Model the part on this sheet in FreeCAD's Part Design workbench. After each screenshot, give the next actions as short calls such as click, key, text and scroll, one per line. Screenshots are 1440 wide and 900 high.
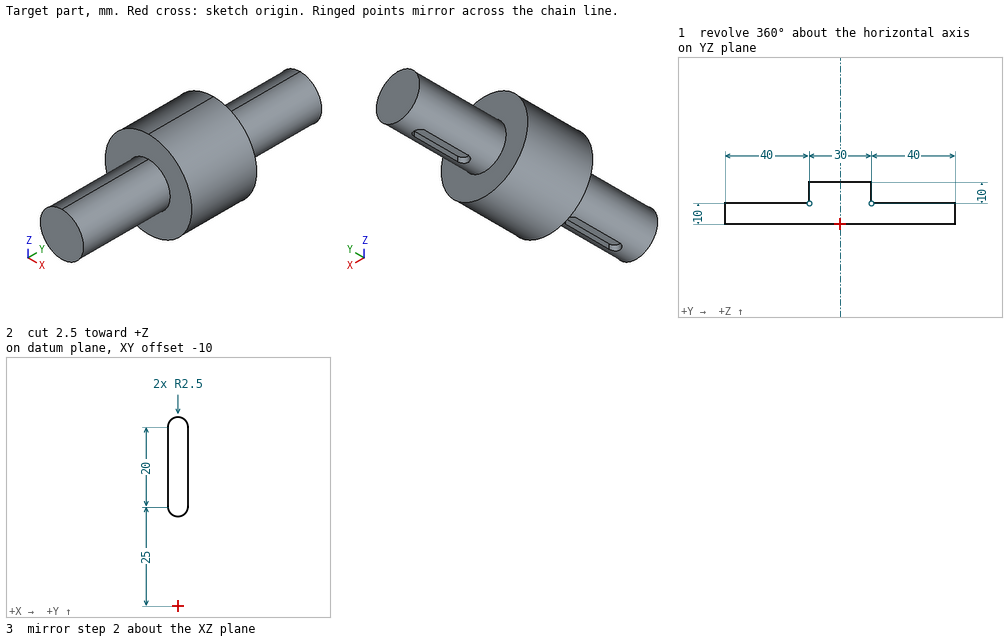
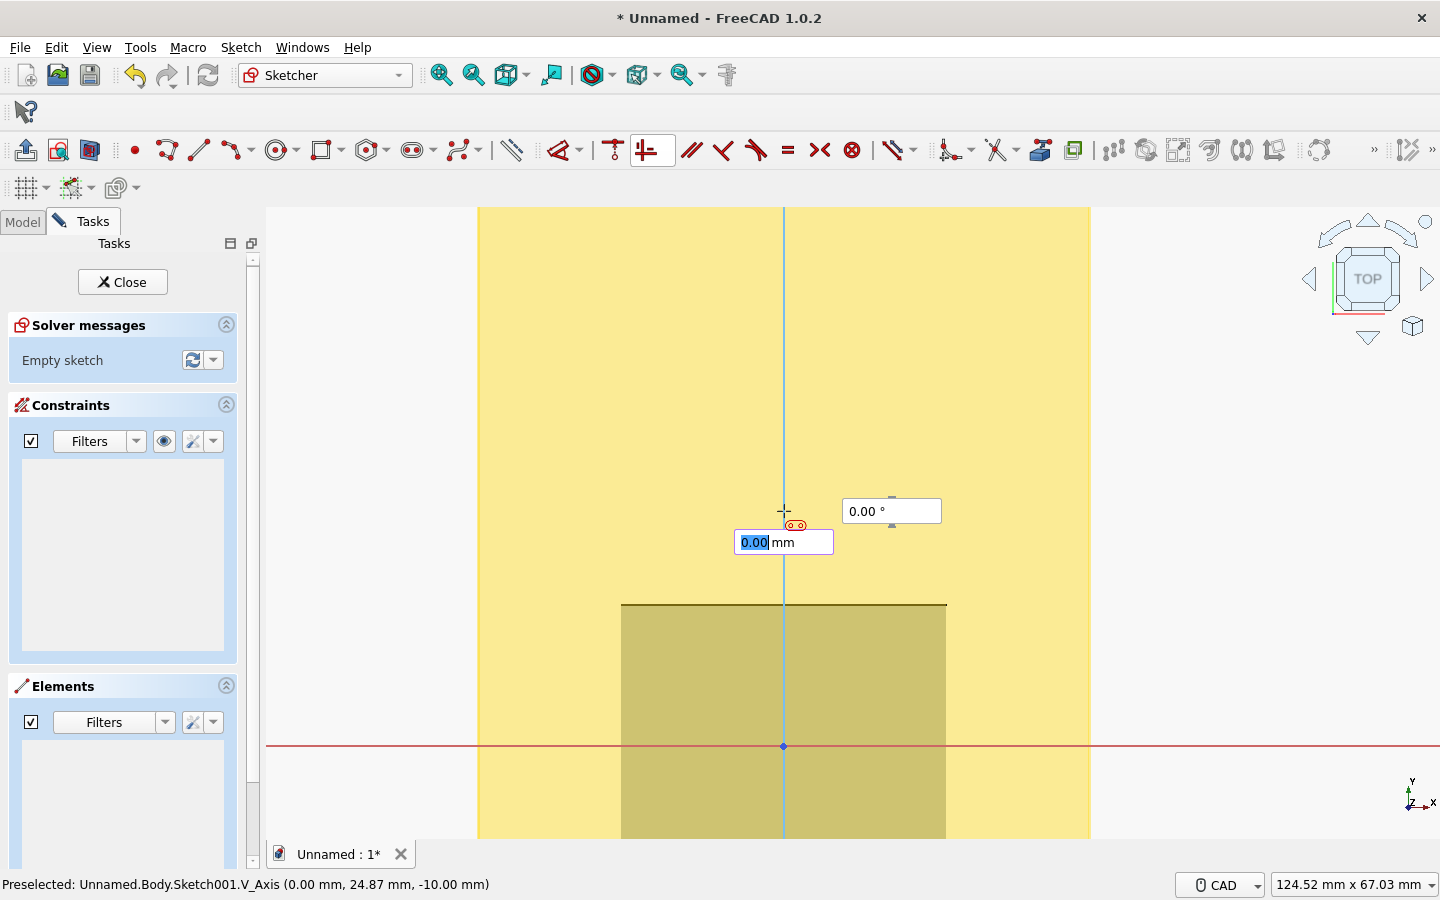
click(793, 322)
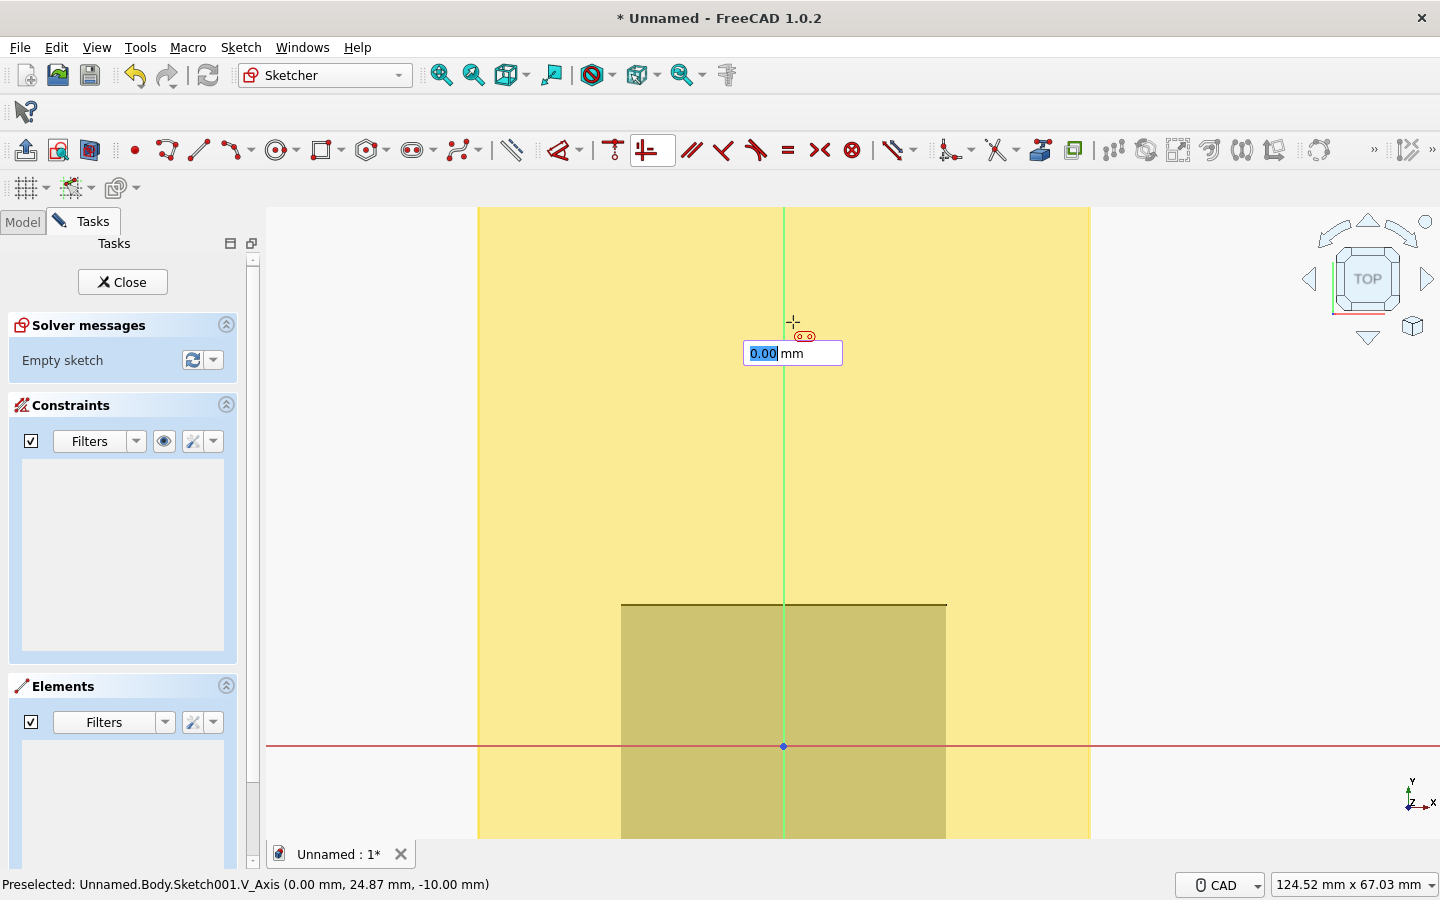
click(760, 416)
key(Escape)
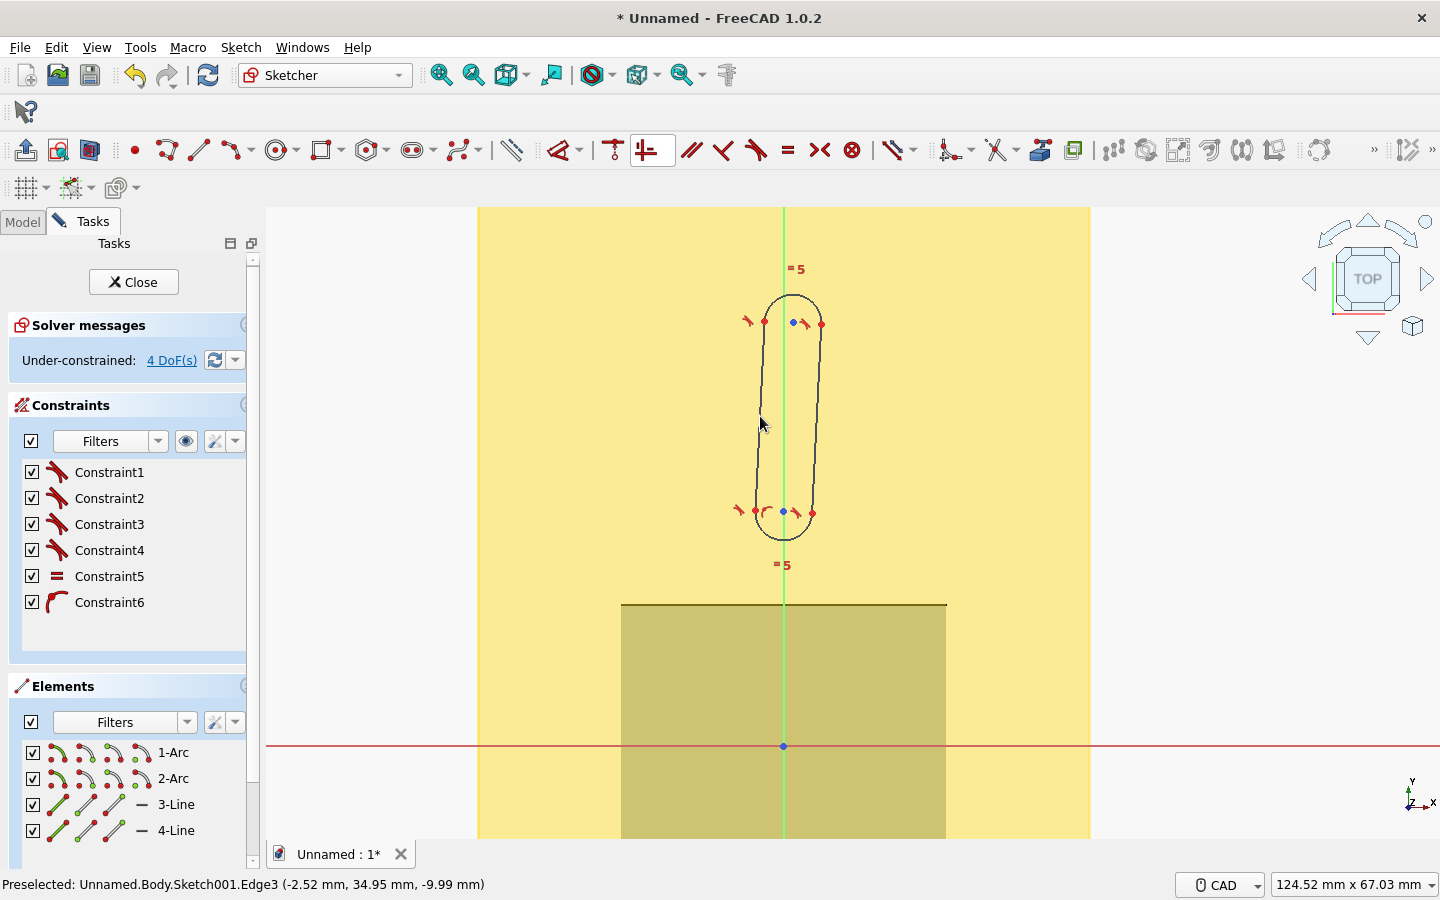
click(758, 454)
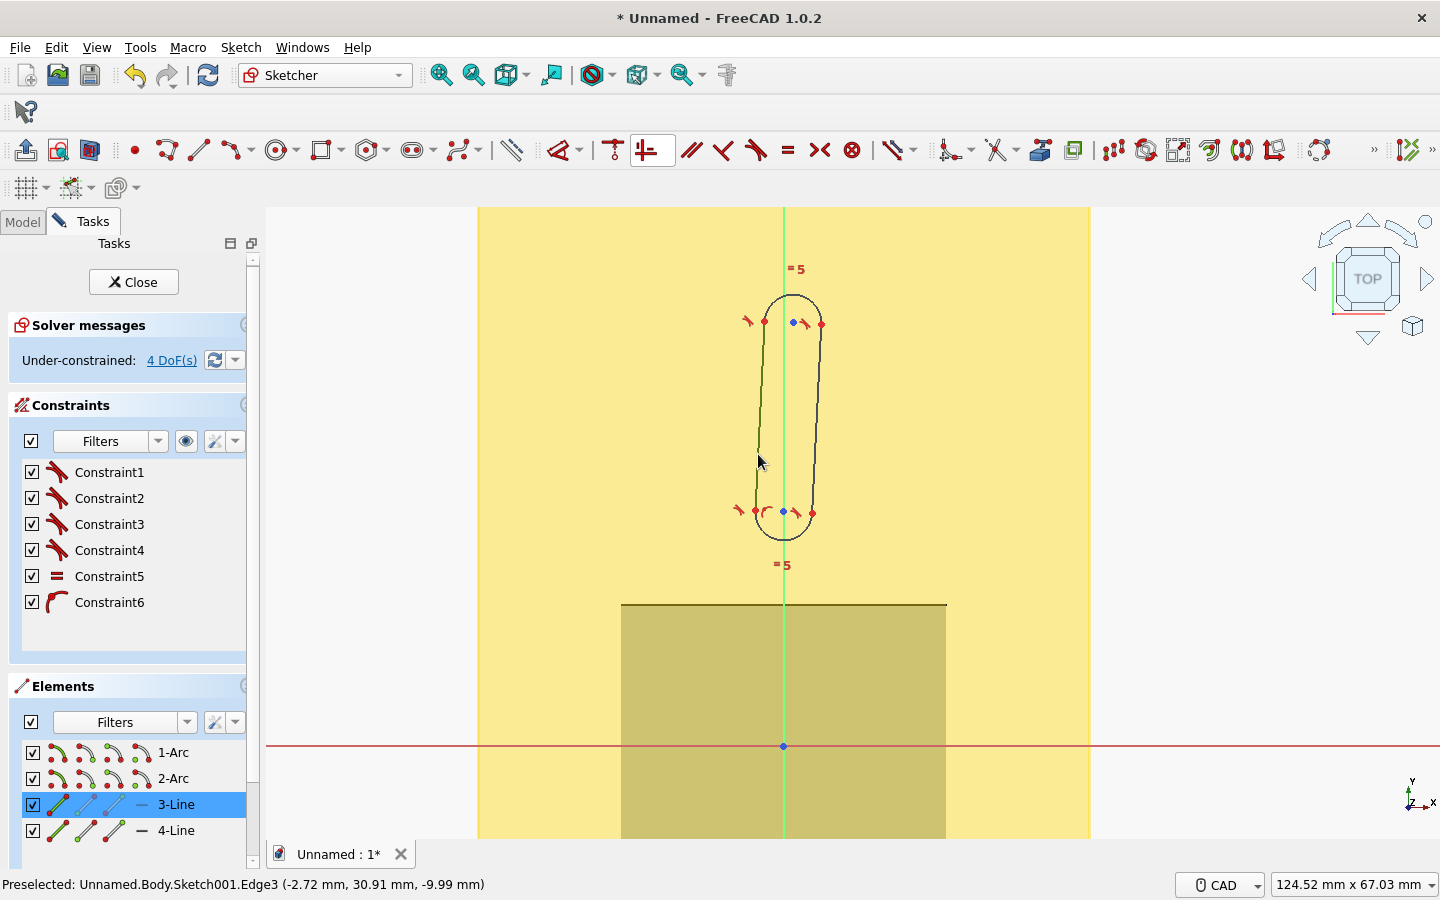
click(670, 150)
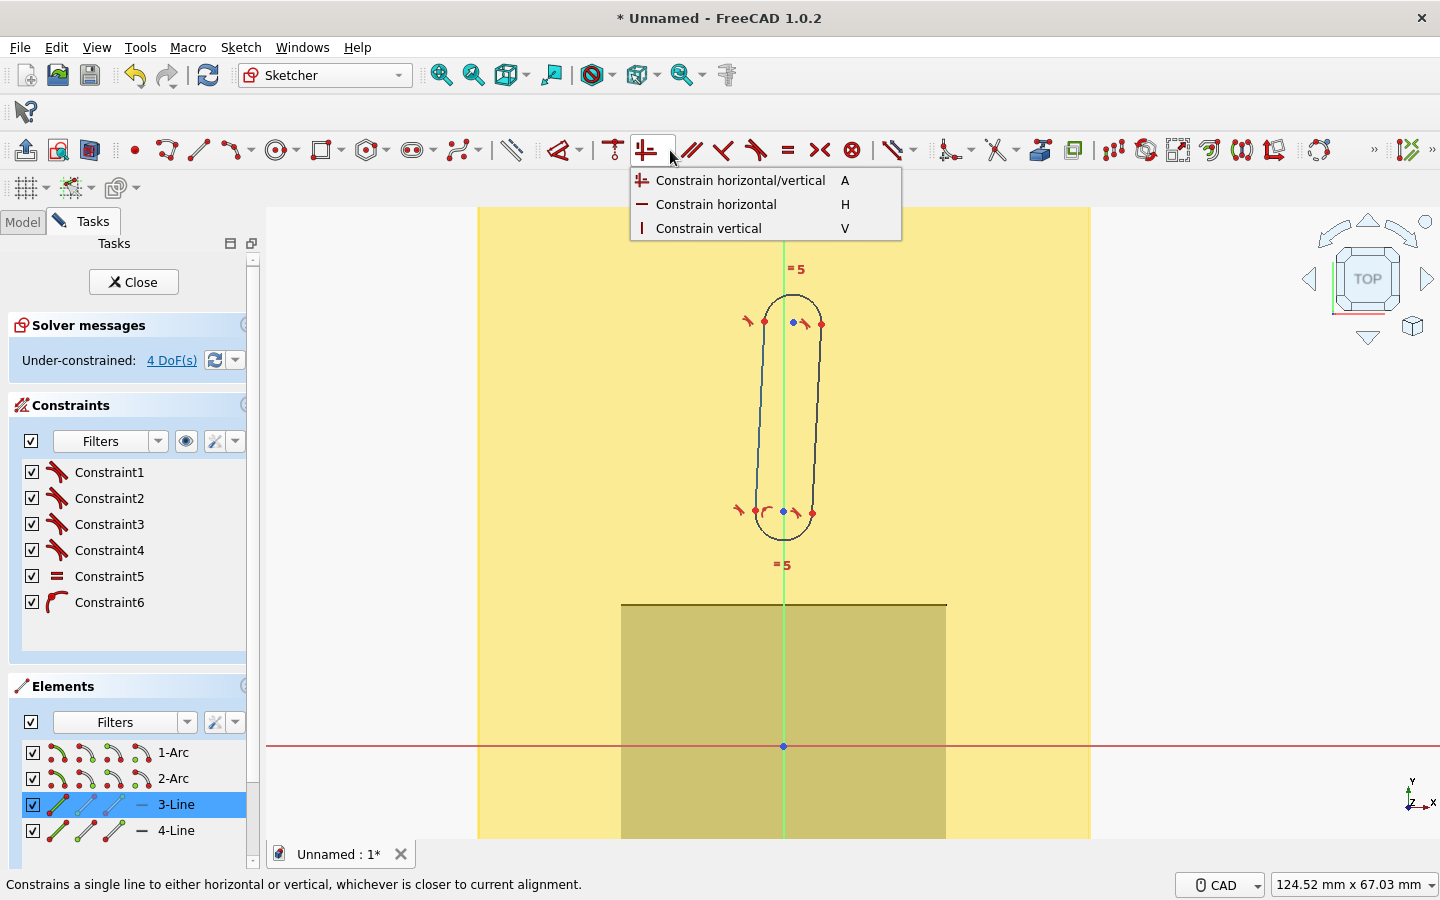
click(766, 228)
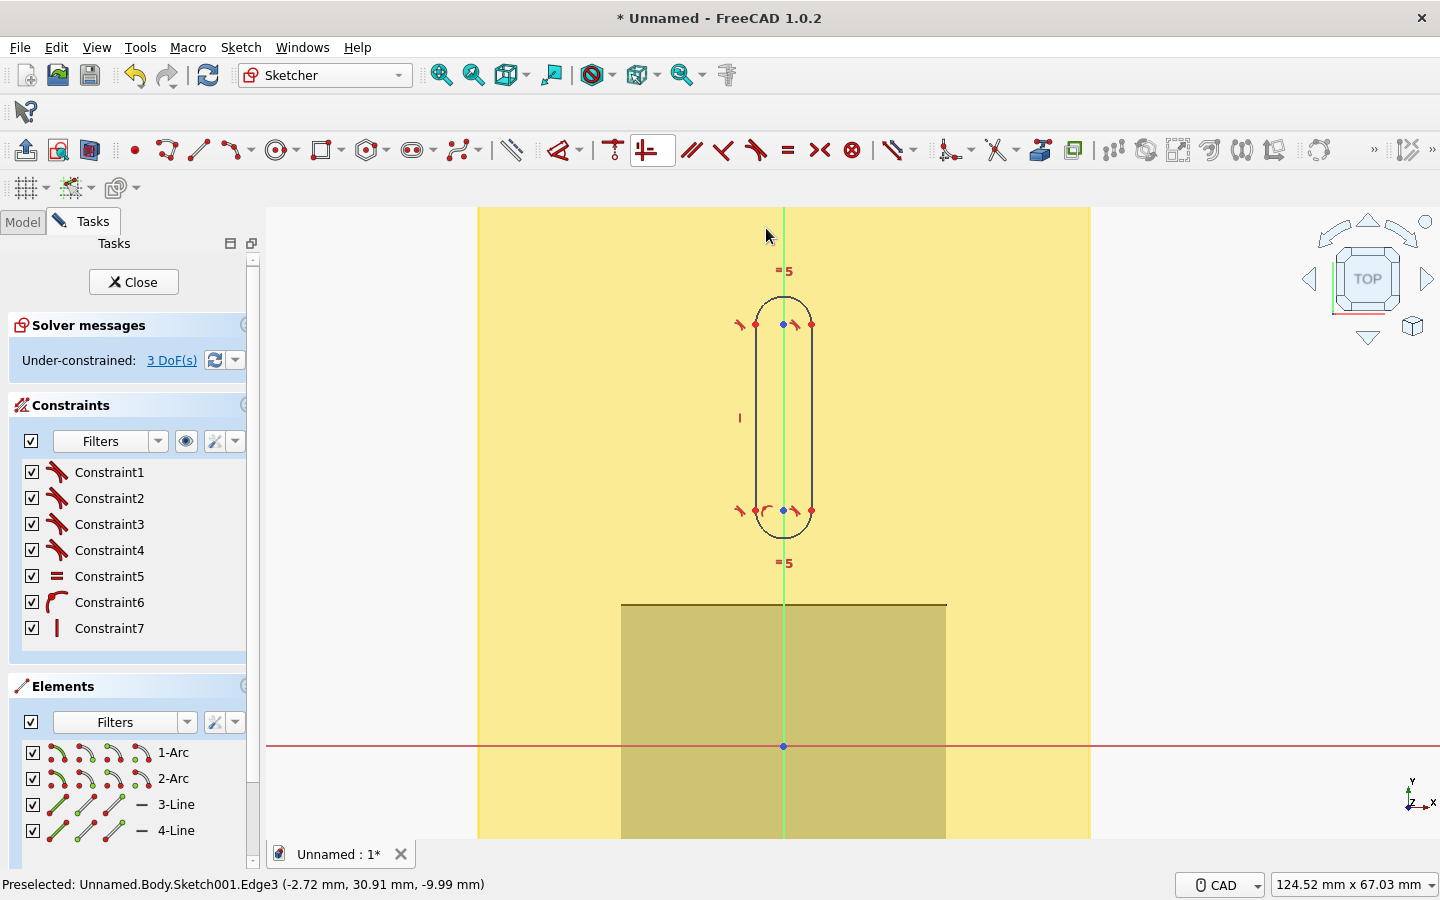
click(558, 150)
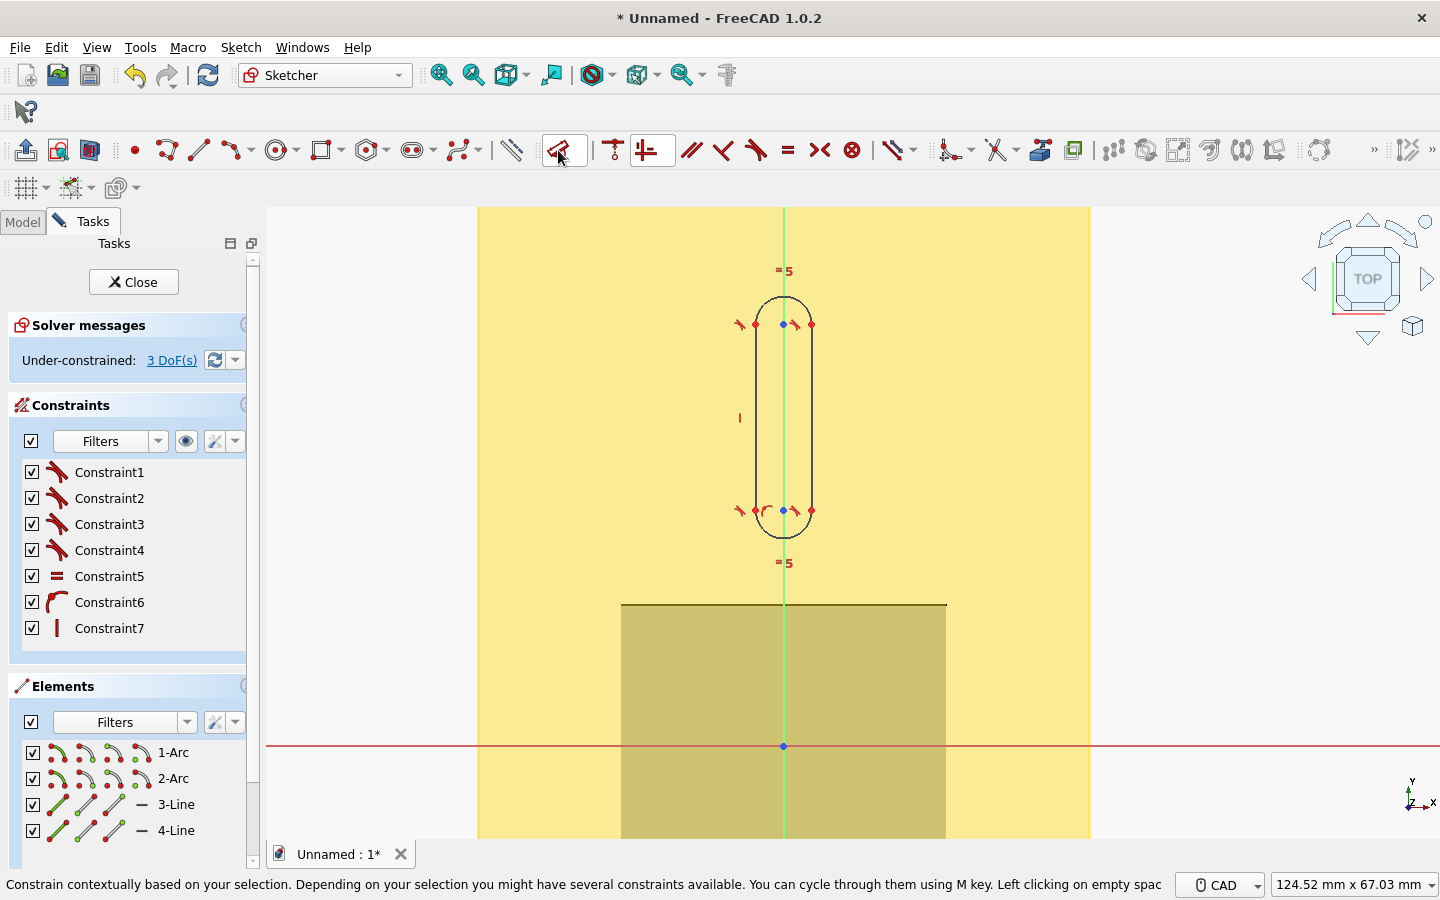
scroll(767, 533, up, 3)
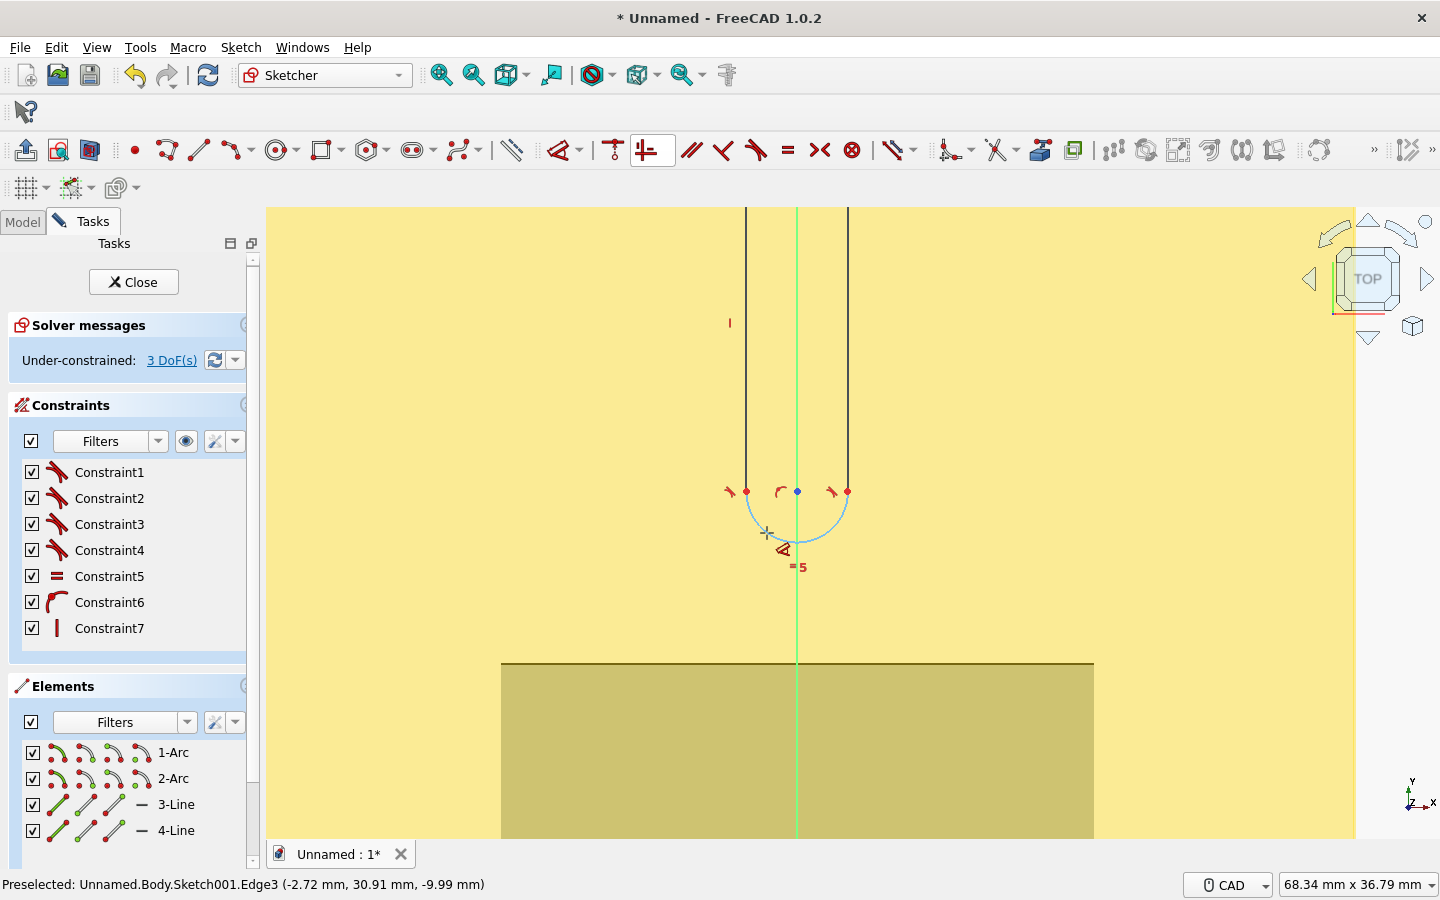
click(767, 533)
click(748, 559)